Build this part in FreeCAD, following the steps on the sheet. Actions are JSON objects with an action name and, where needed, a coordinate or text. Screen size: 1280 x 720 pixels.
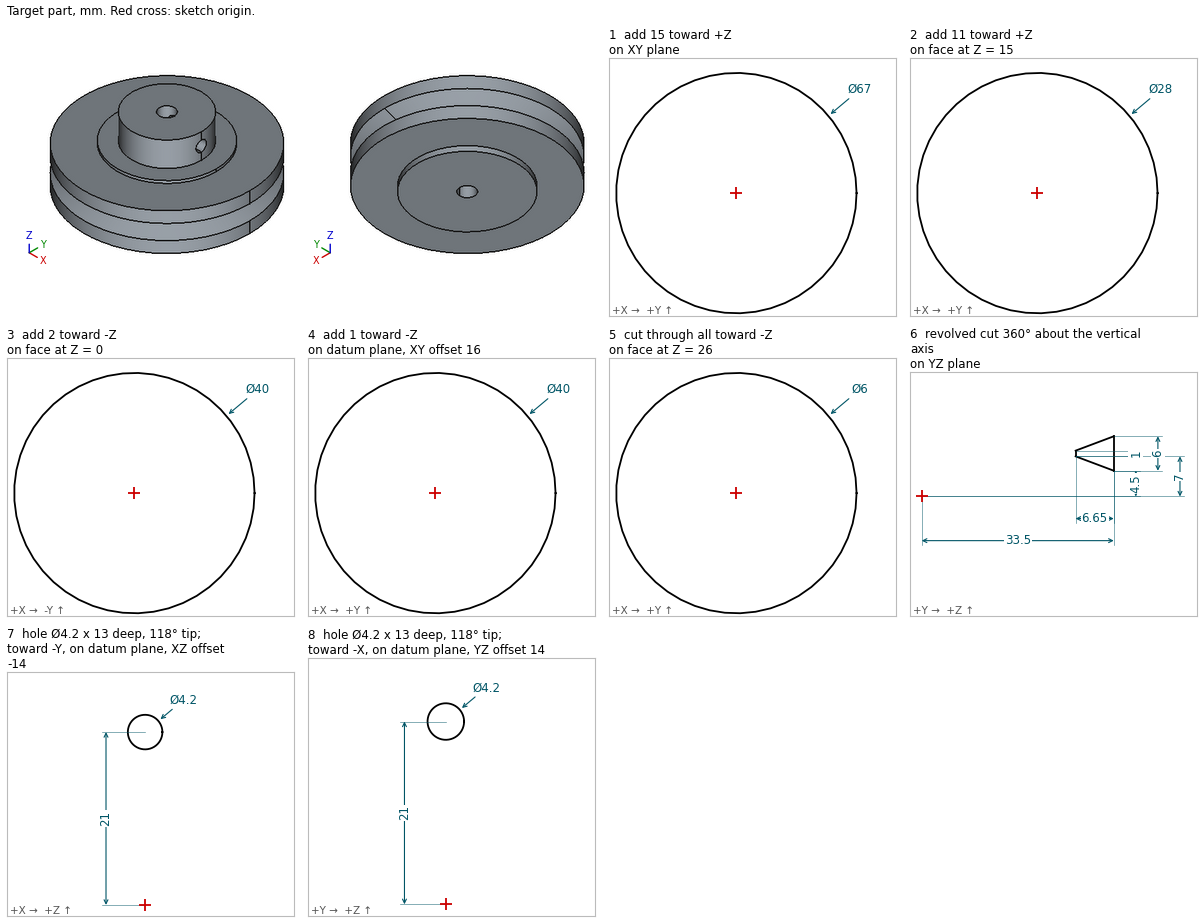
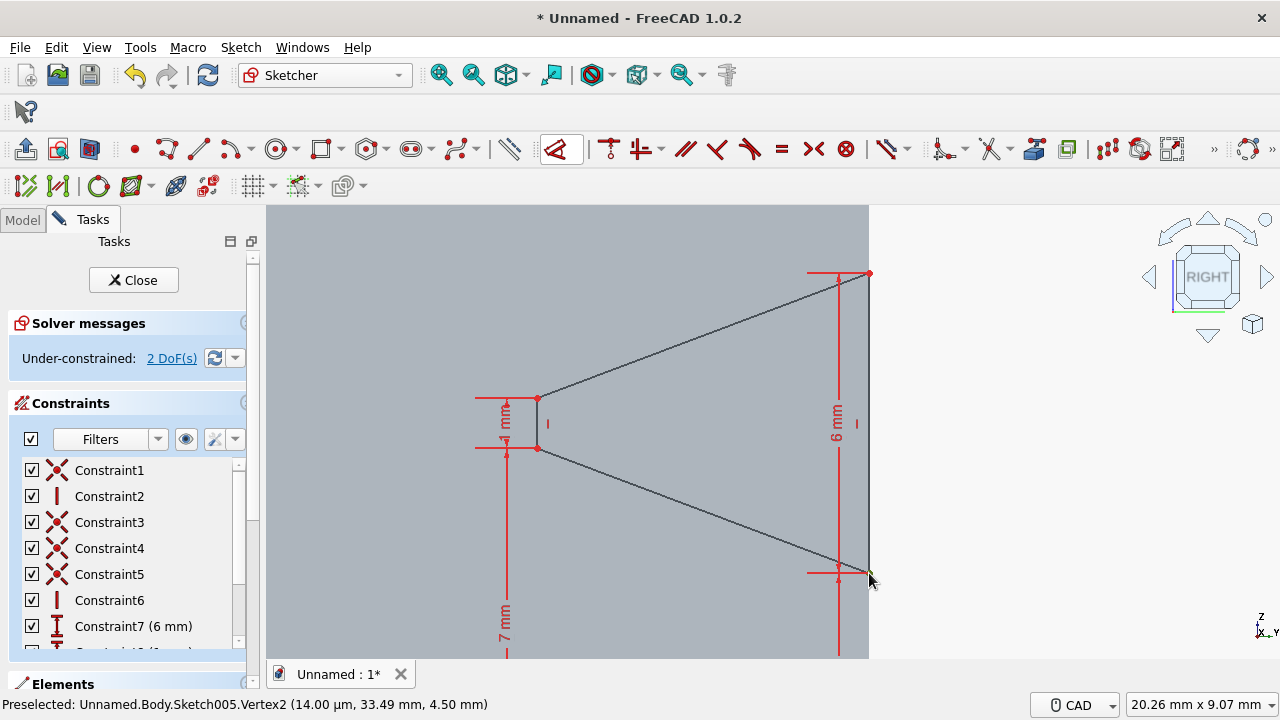
{"action": "key", "text": "l"}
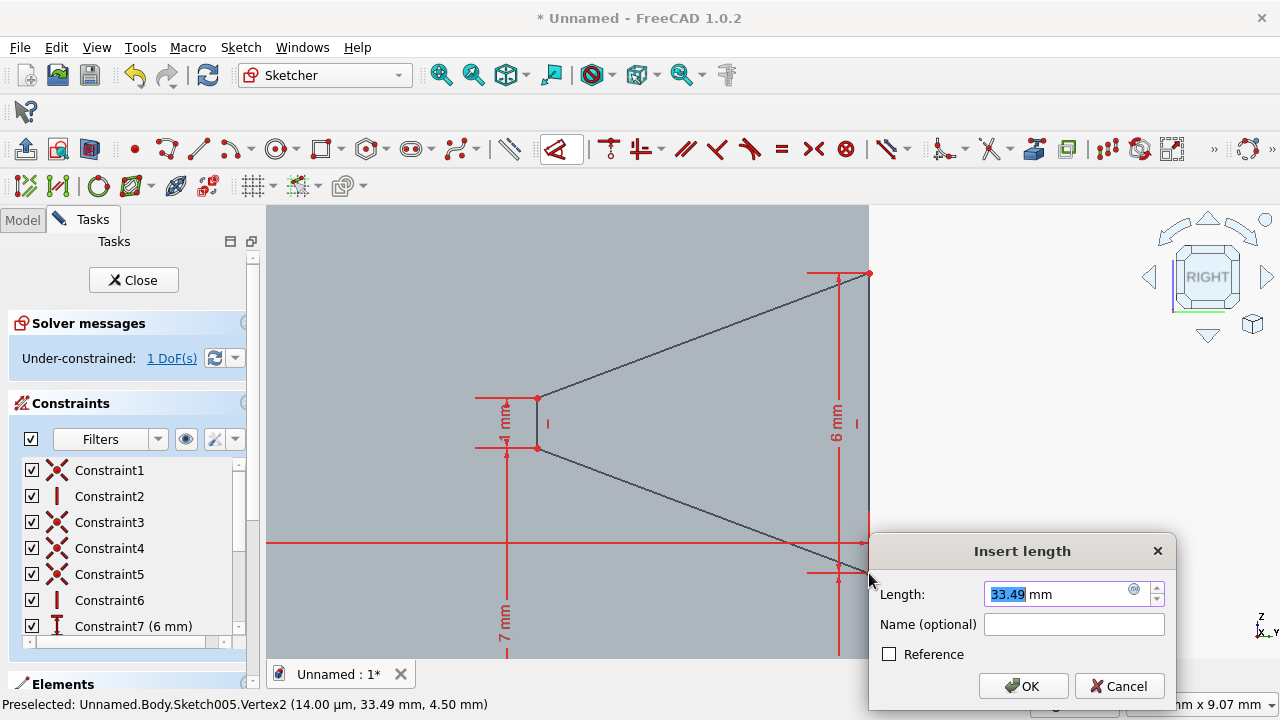
{"action": "type", "text": "33.5"}
{"action": "key", "text": "Return"}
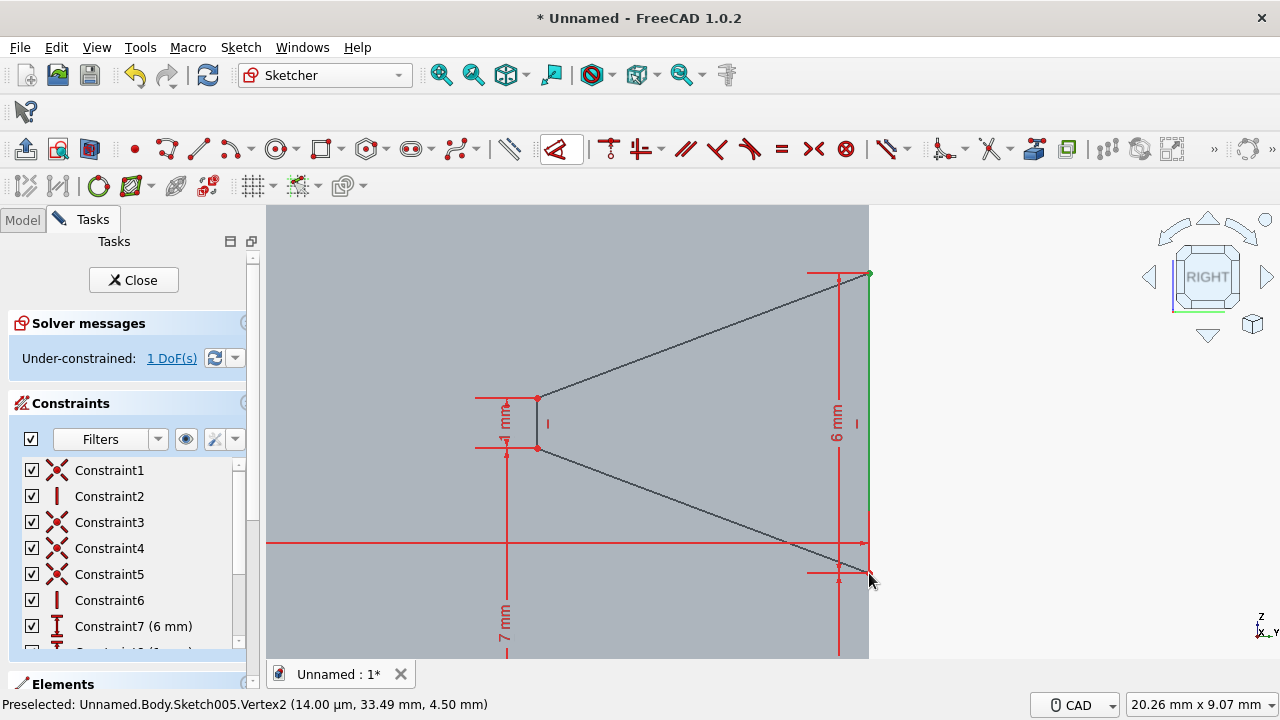
{"action": "left_click", "coordinate": [637, 486]}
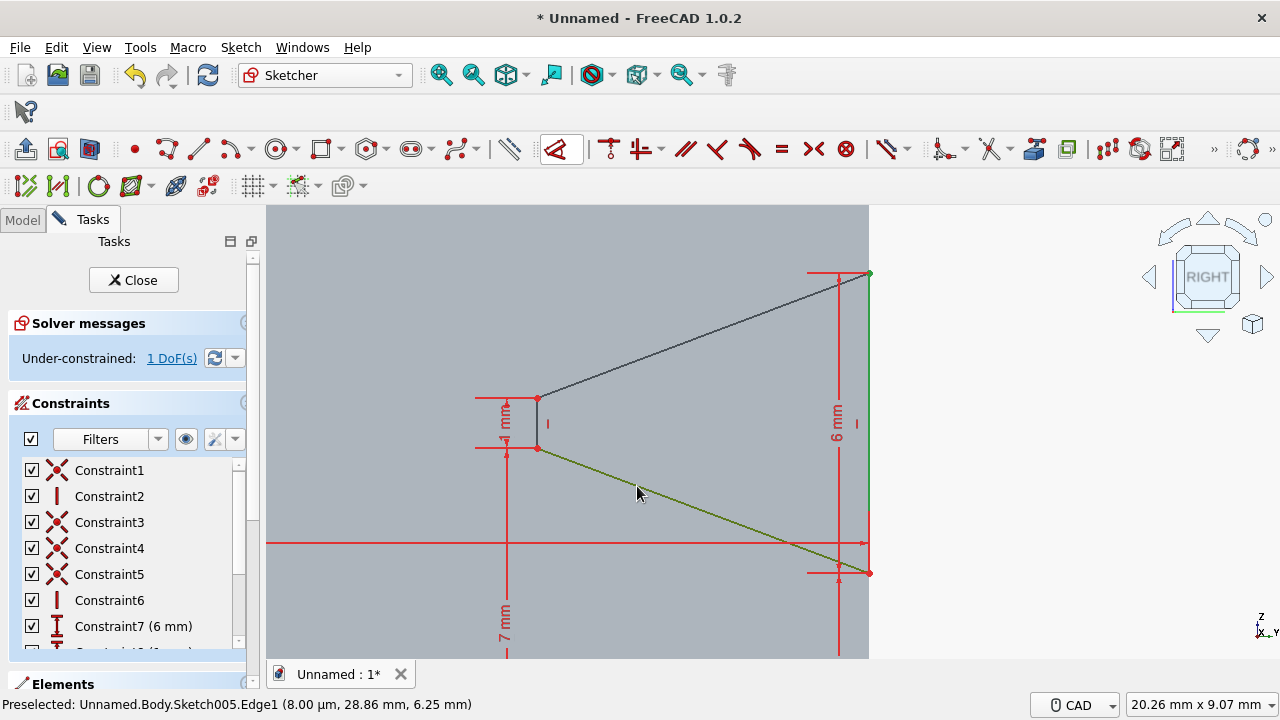
{"action": "key", "text": "l"}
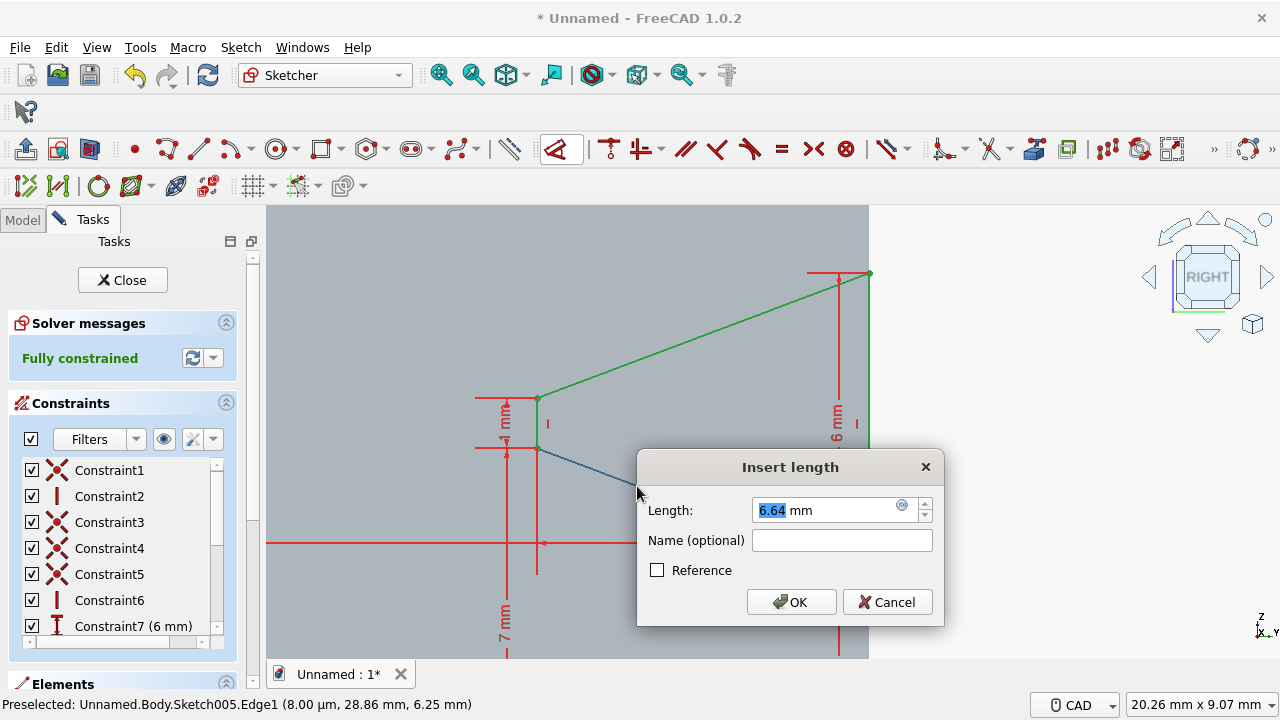
{"action": "type", "text": "6.65"}
{"action": "key", "text": "Return"}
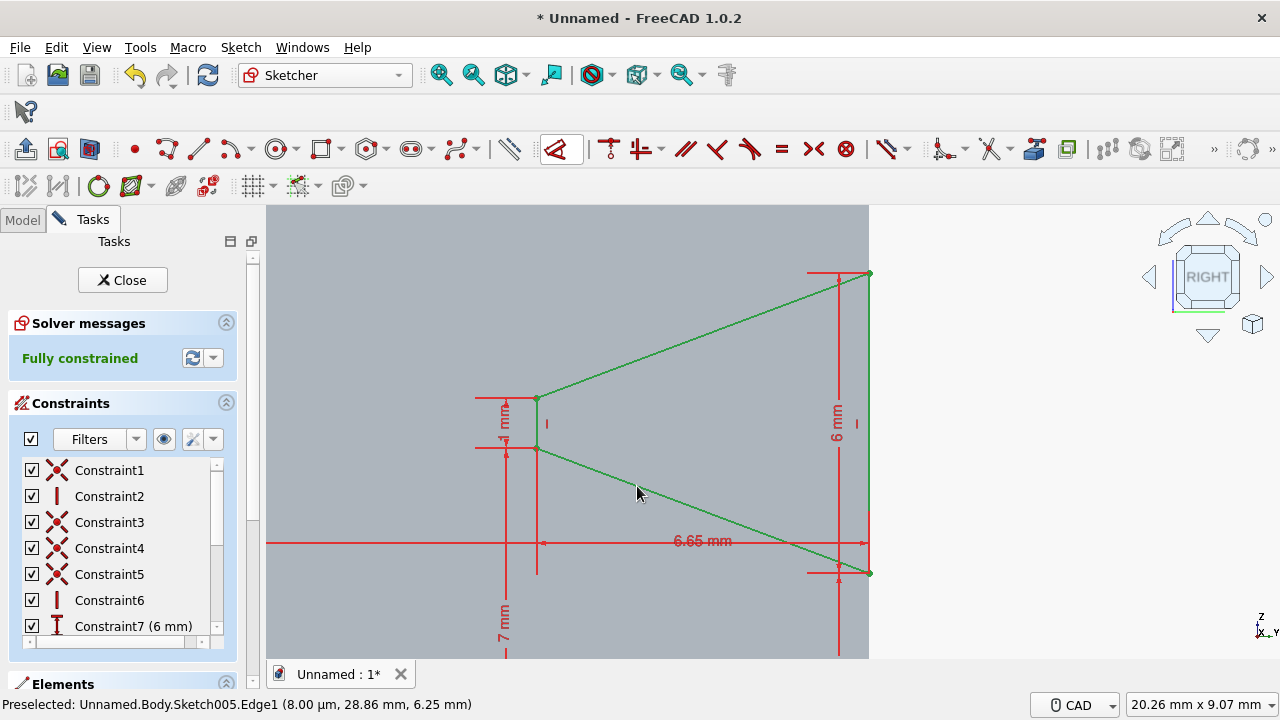
{"action": "left_click", "coordinate": [123, 280]}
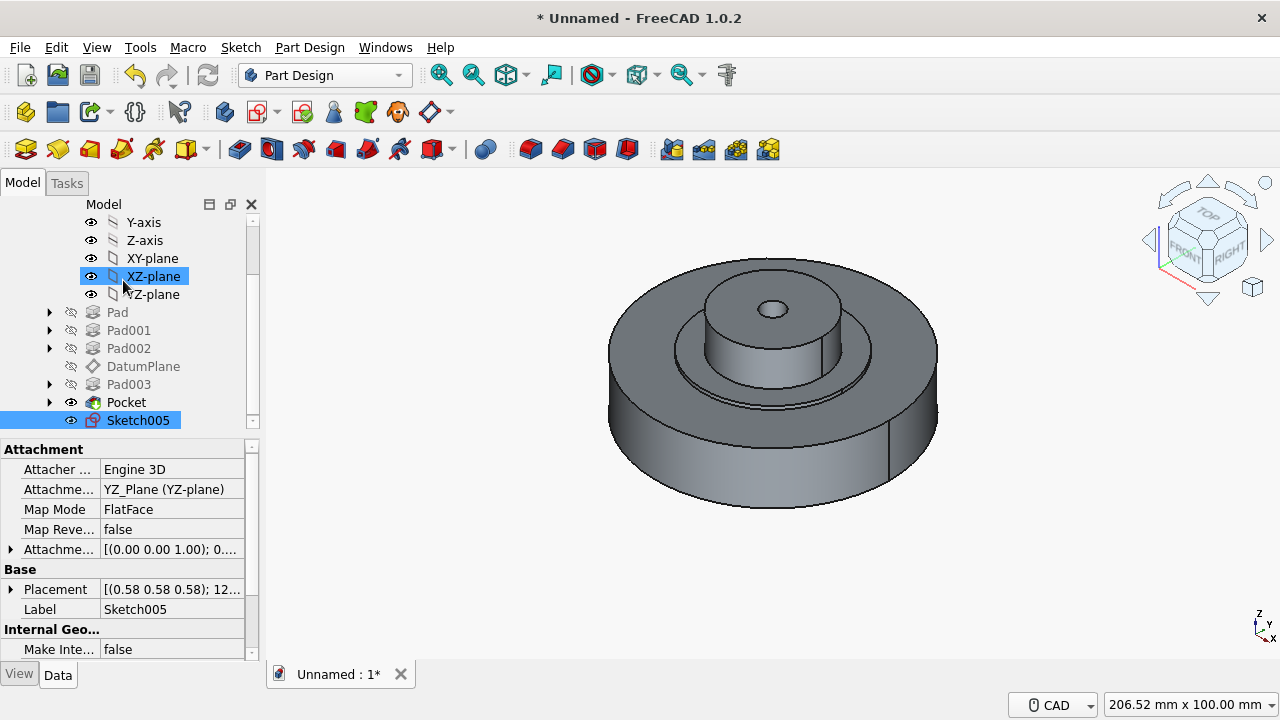
{"action": "left_click", "coordinate": [304, 150]}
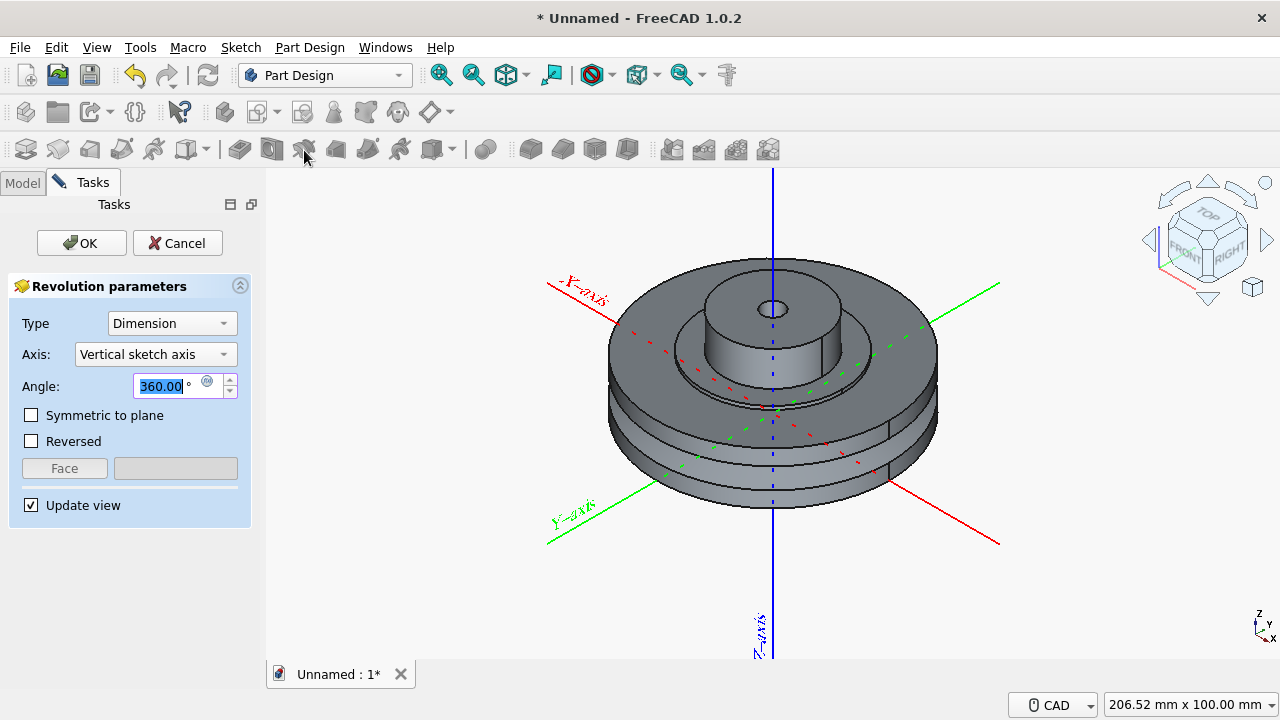
{"action": "left_click", "coordinate": [82, 243]}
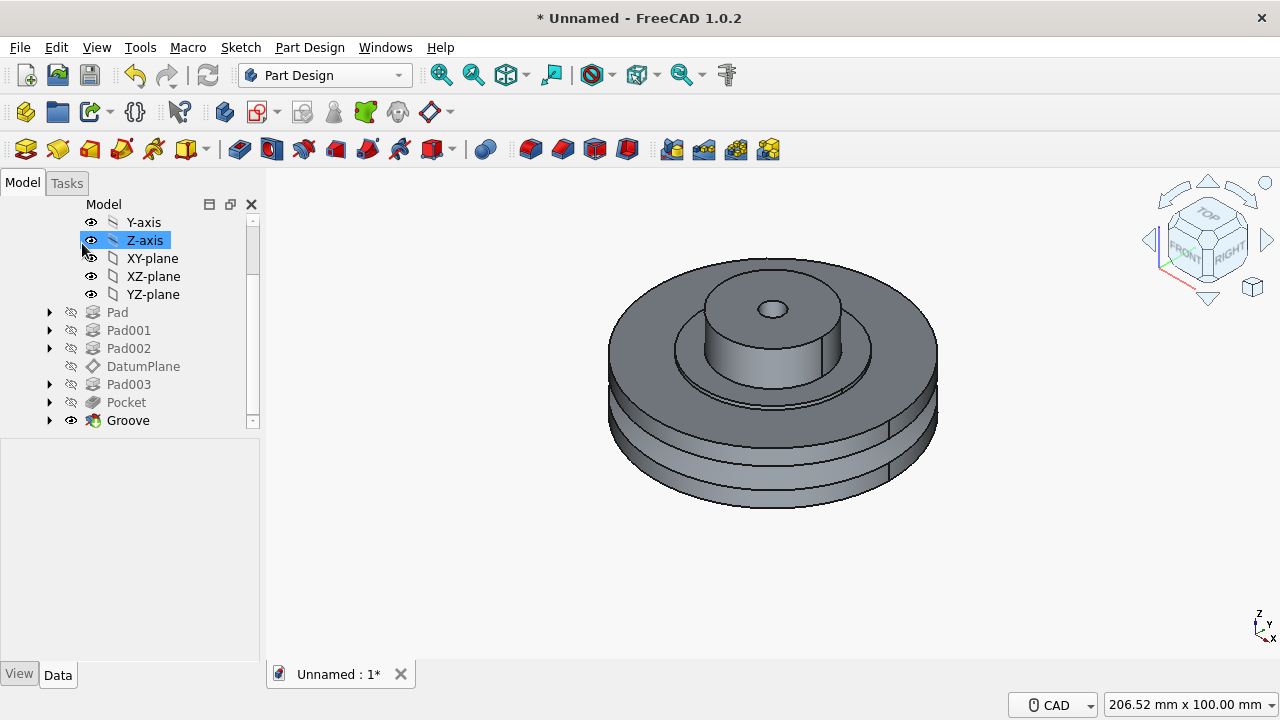
{"action": "scroll", "coordinate": [160, 326], "scroll_direction": "down", "scroll_amount": 3}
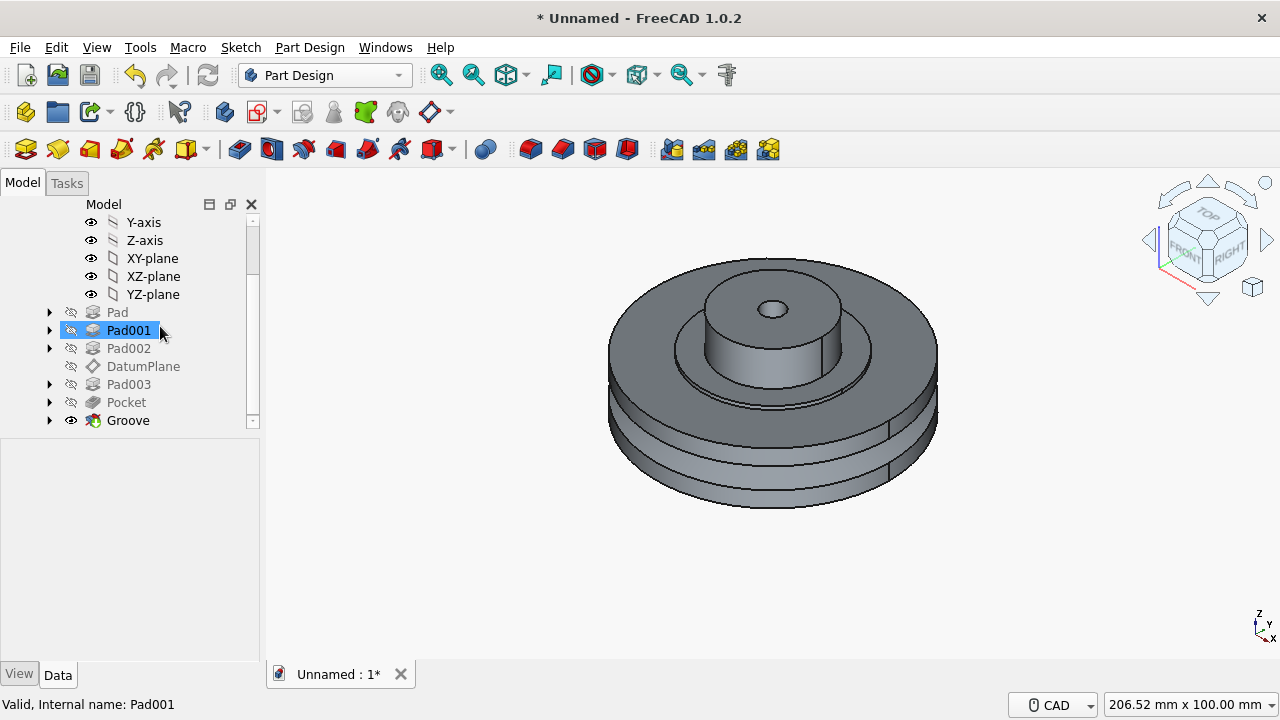
{"action": "scroll", "coordinate": [160, 326], "scroll_direction": "up", "scroll_amount": 15}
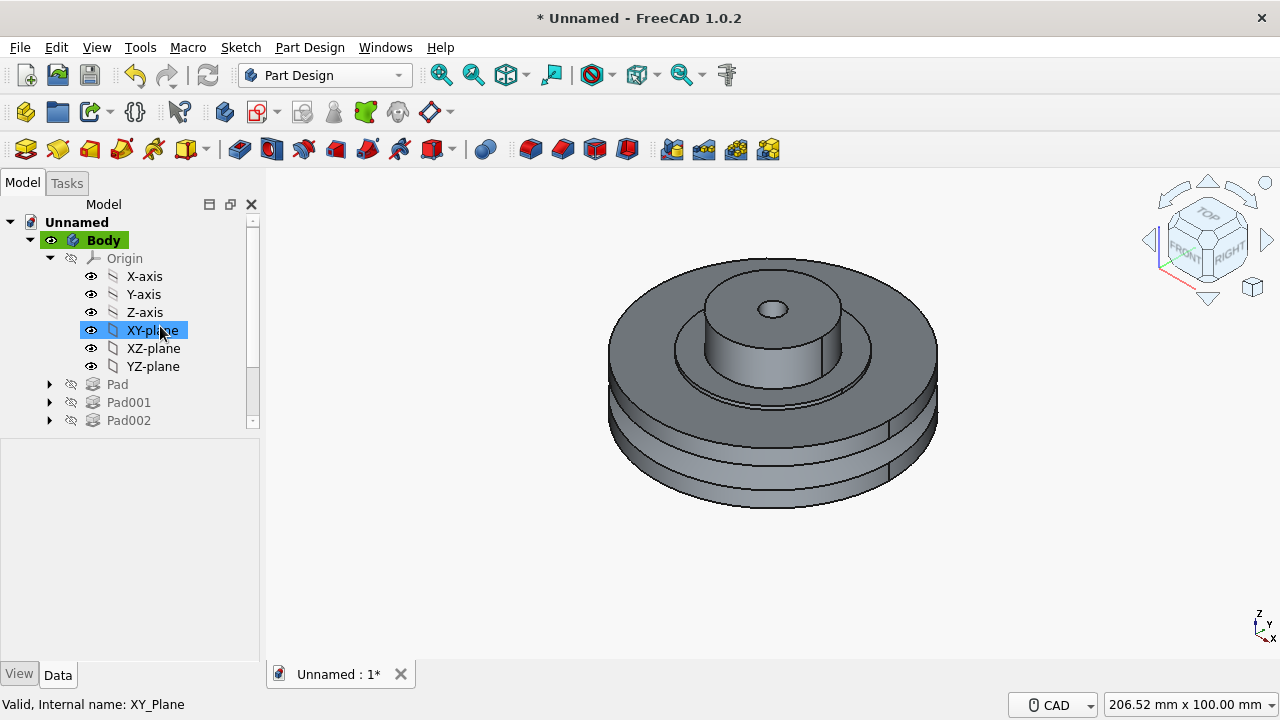
{"action": "left_click", "coordinate": [136, 348]}